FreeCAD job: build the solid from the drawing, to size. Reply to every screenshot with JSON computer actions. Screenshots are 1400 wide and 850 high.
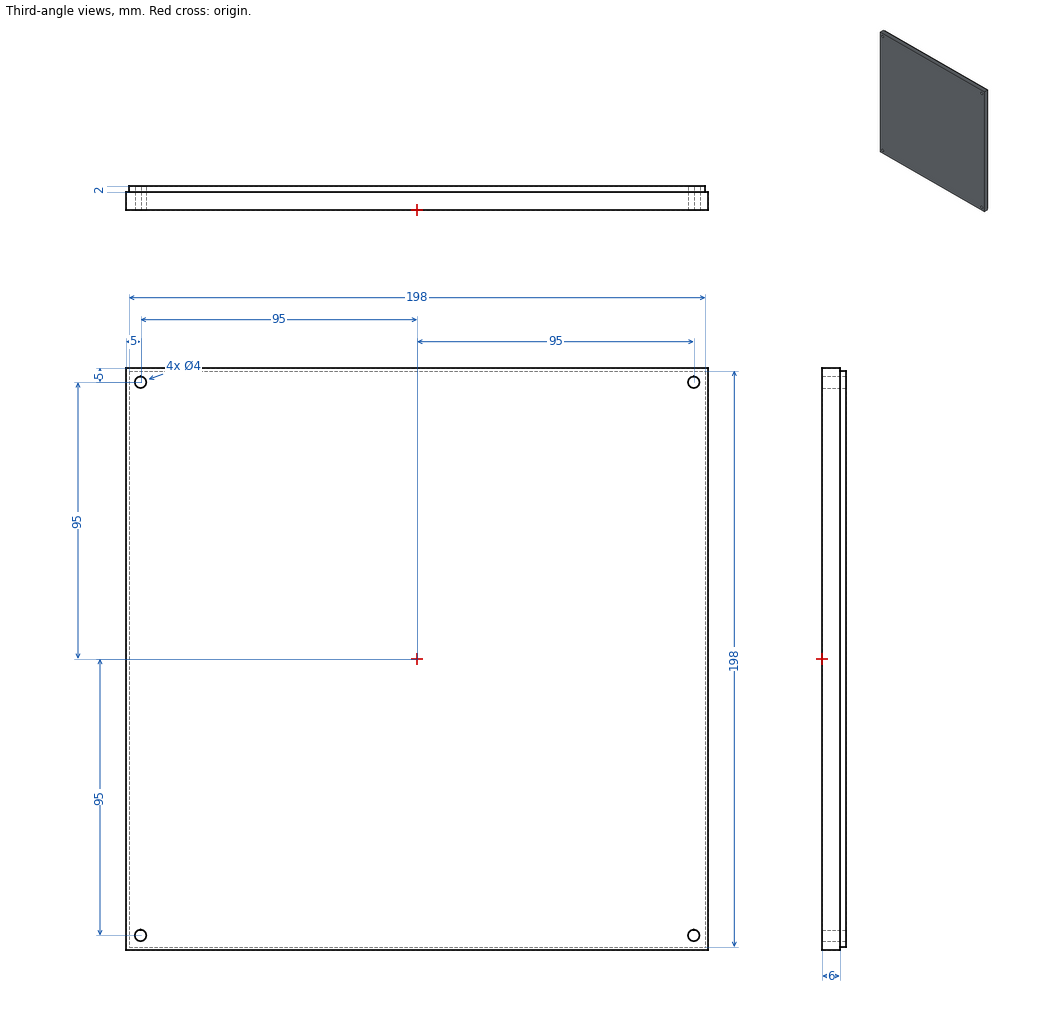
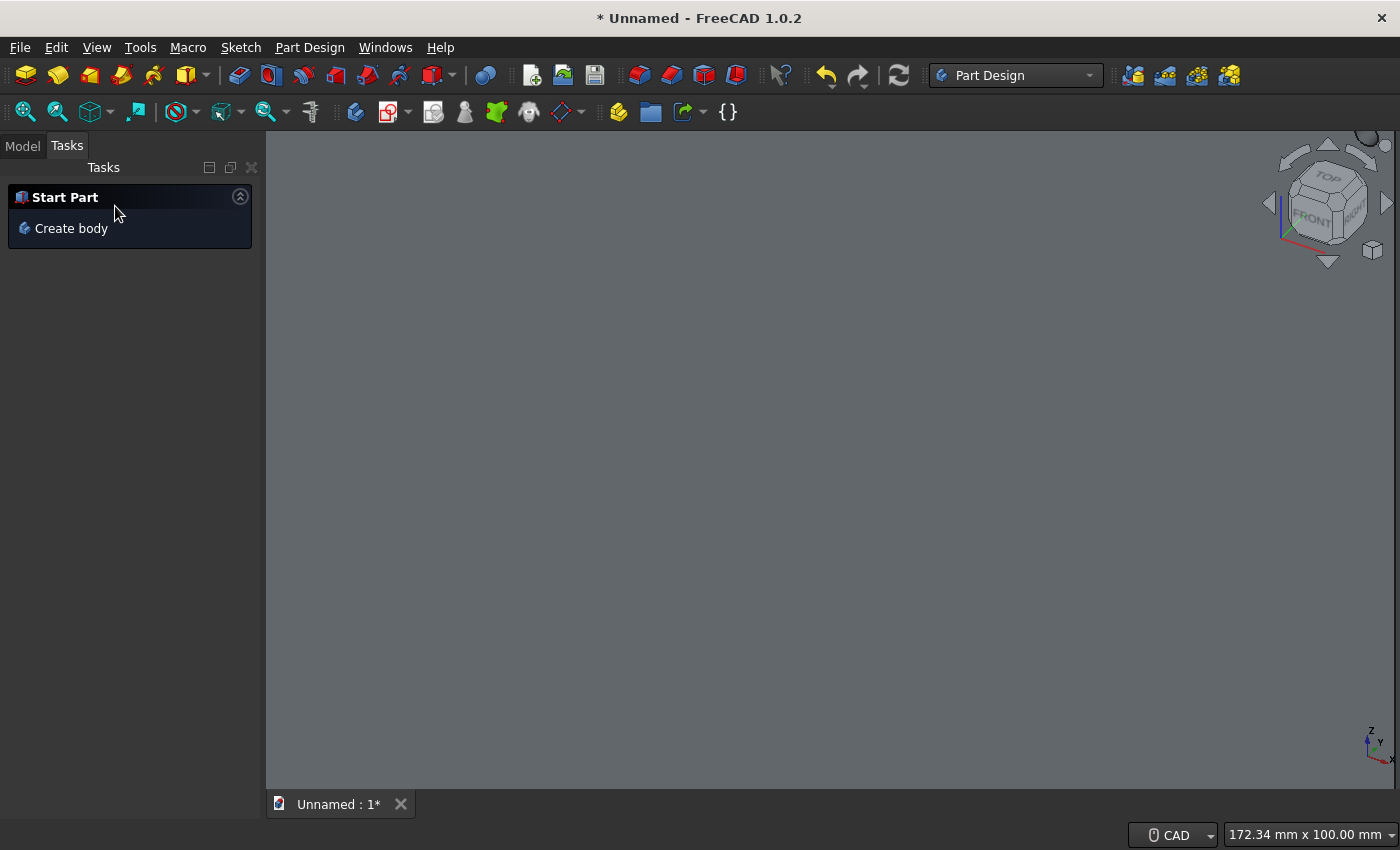
{"action": "left_click", "coordinate": [26, 112]}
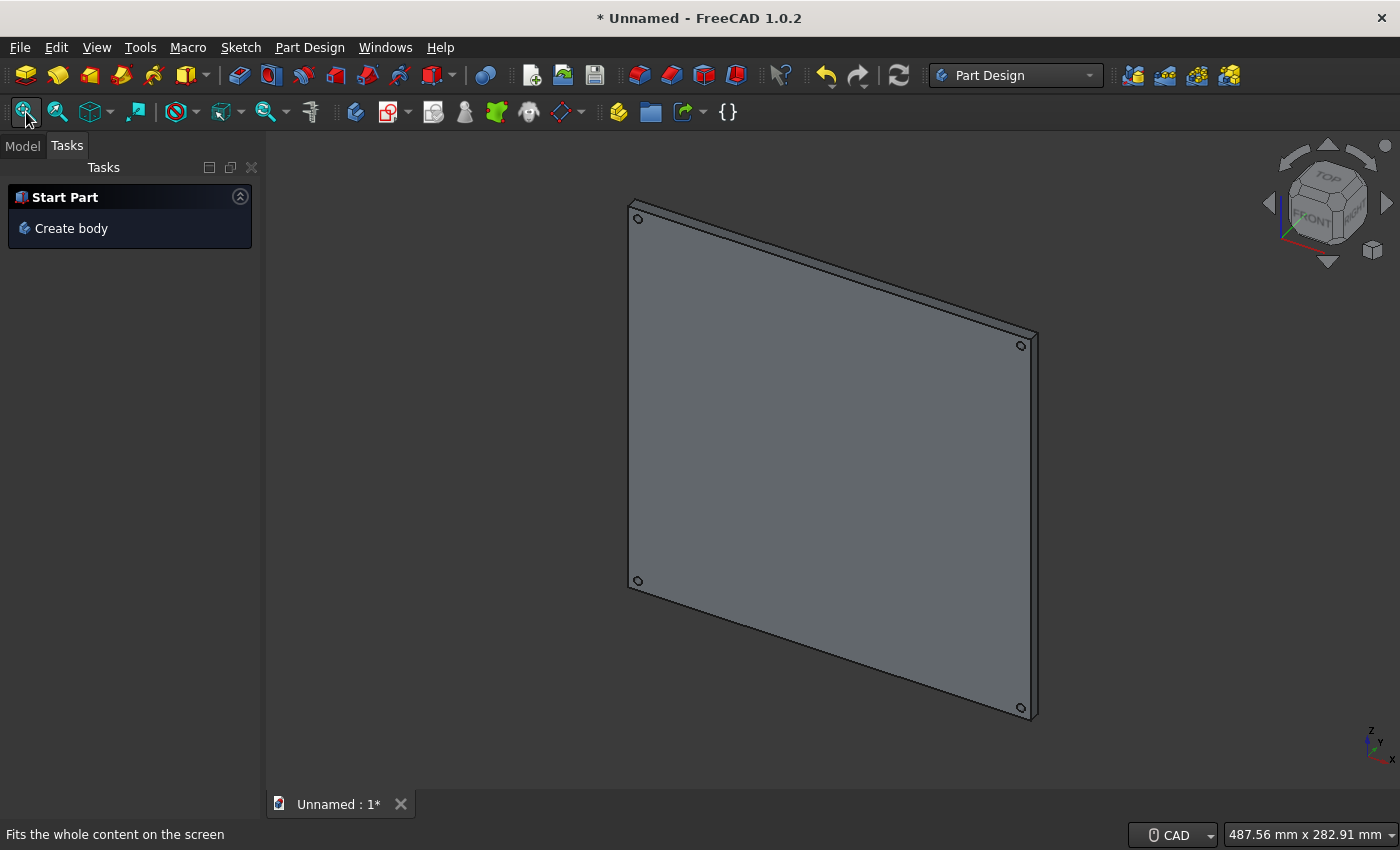
{"action": "key", "text": "4"}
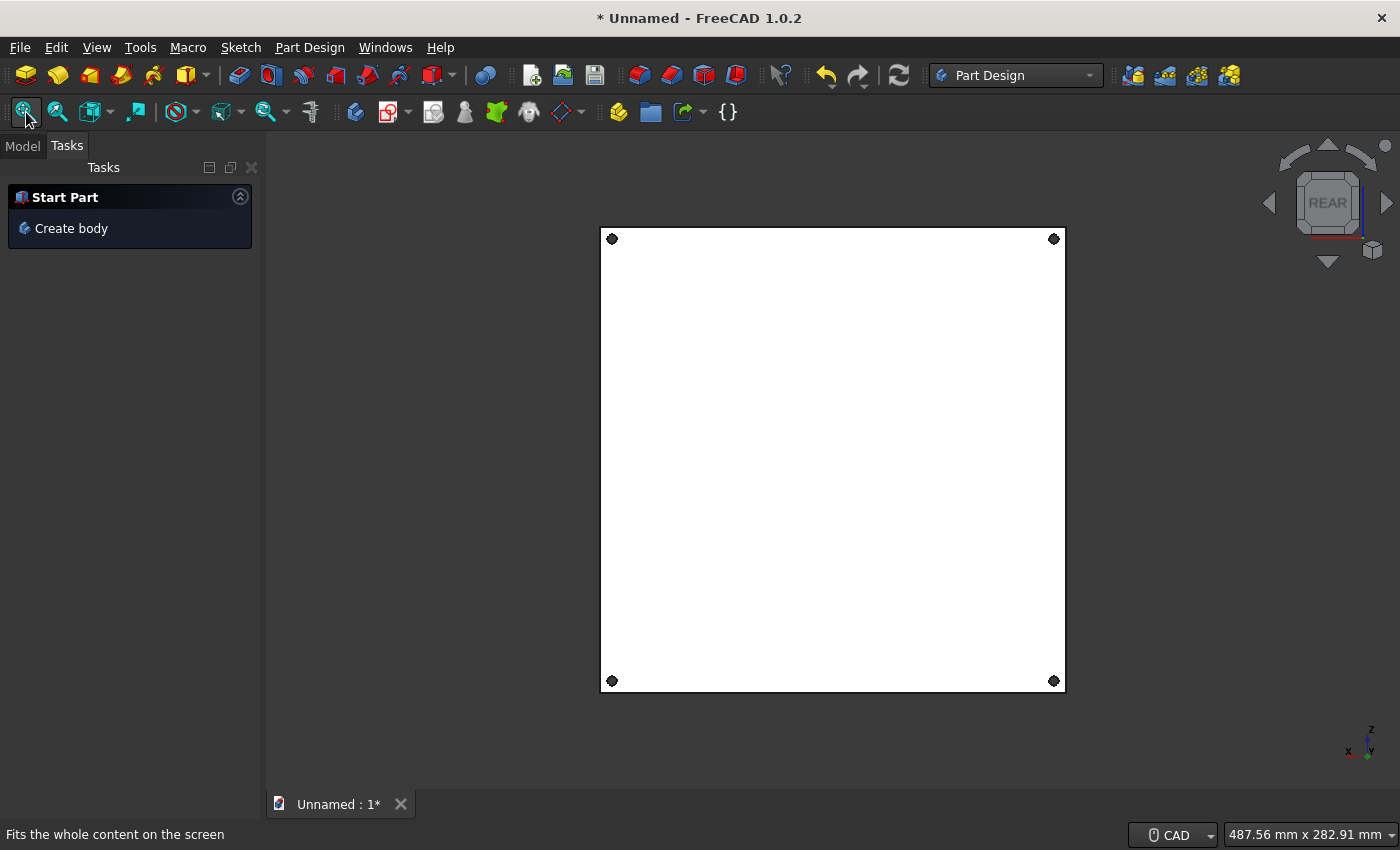
{"action": "left_click", "coordinate": [833, 459]}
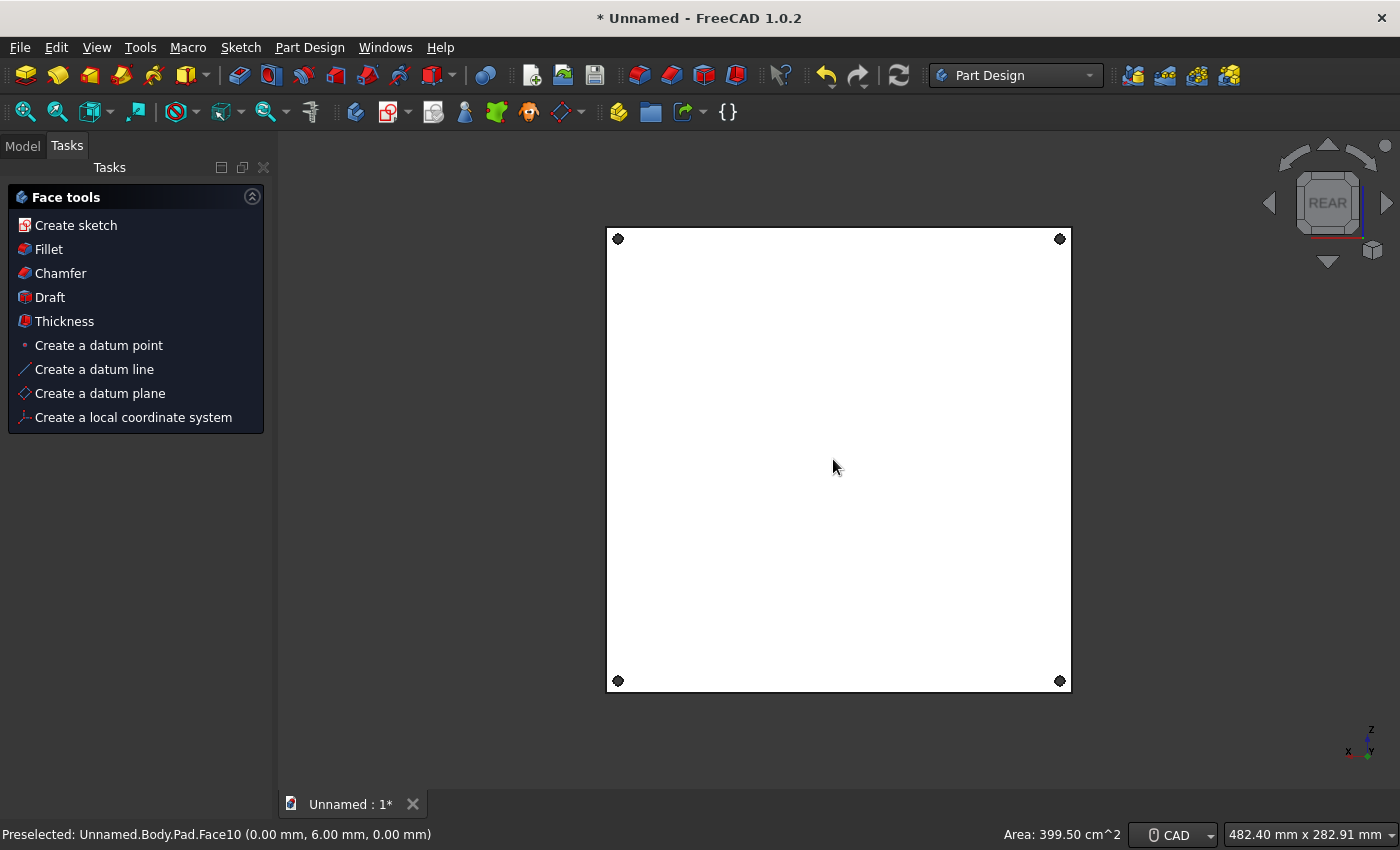
{"action": "left_click", "coordinate": [388, 112]}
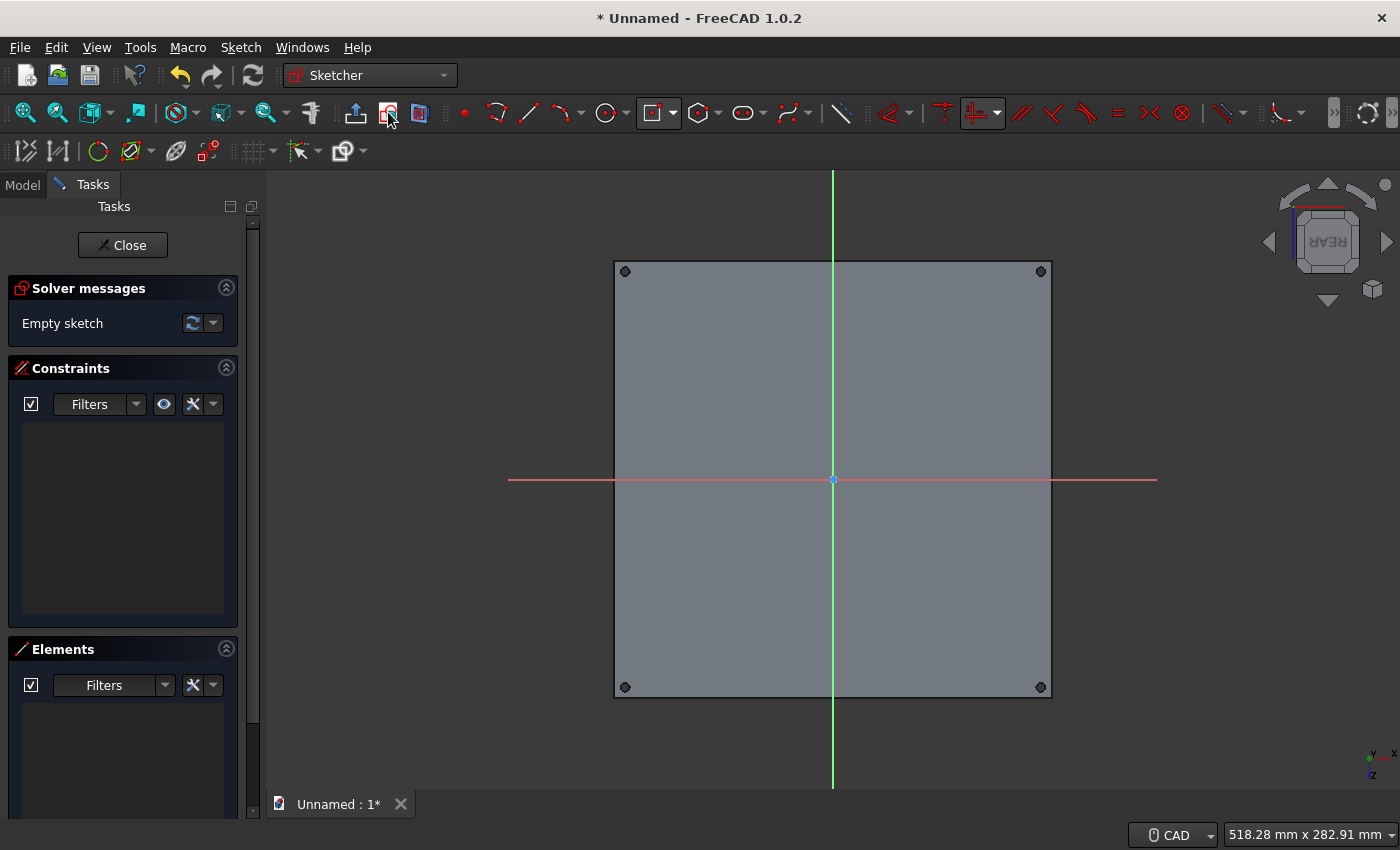
{"action": "left_click", "coordinate": [652, 114]}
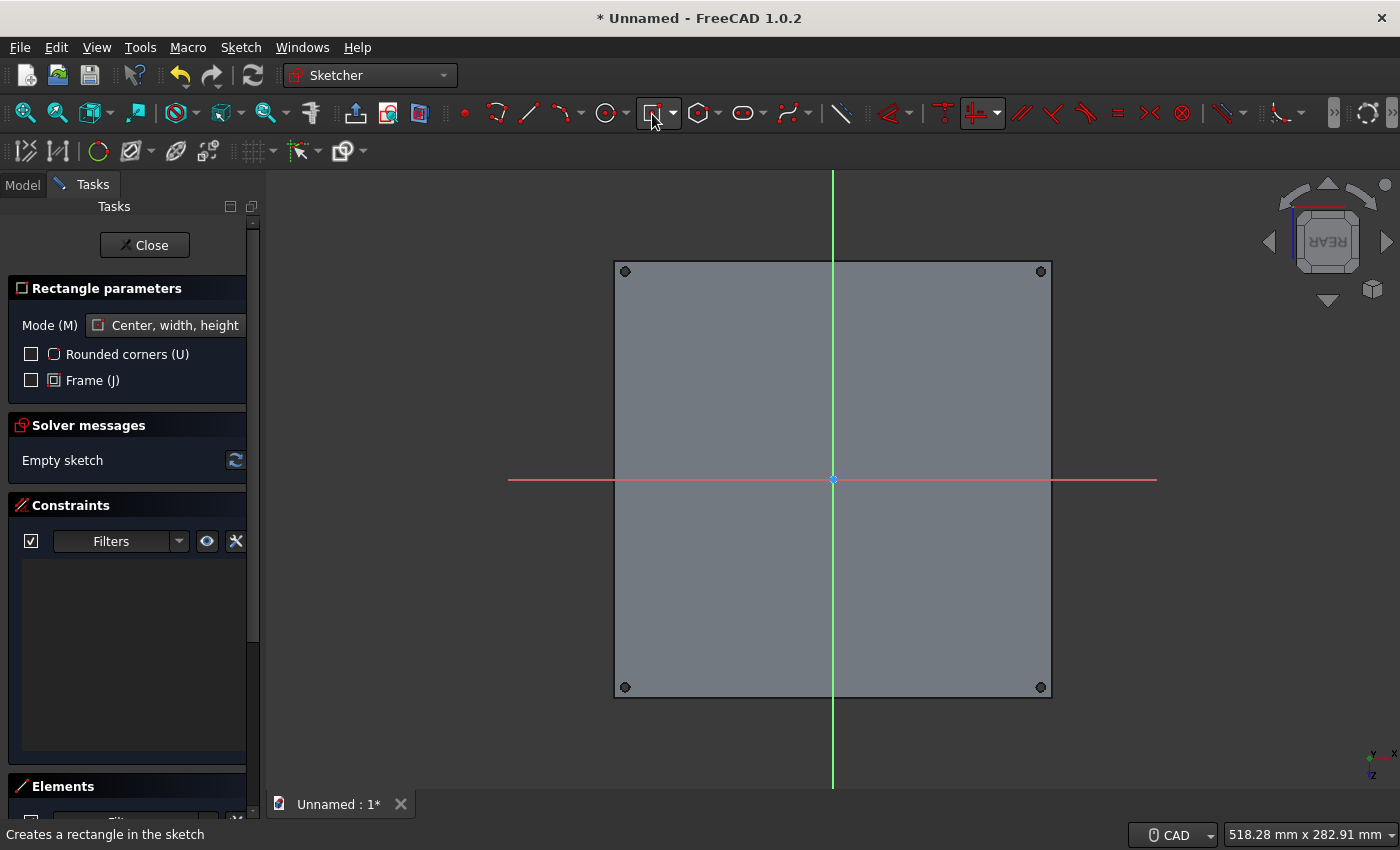
{"action": "left_click", "coordinate": [833, 480]}
{"action": "left_click", "coordinate": [1050, 263]}
{"action": "key", "text": "Escape"}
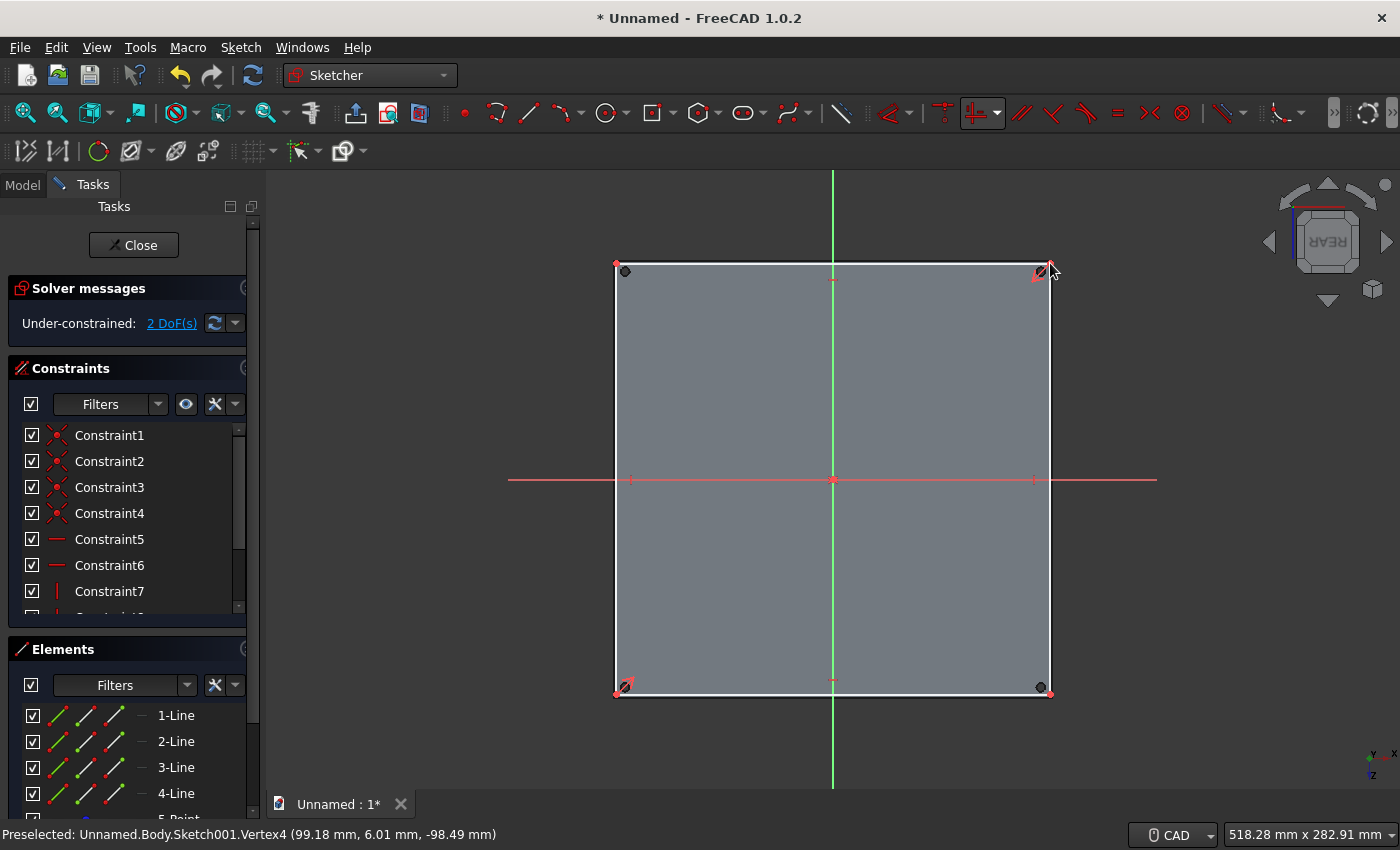
{"action": "left_click", "coordinate": [888, 114]}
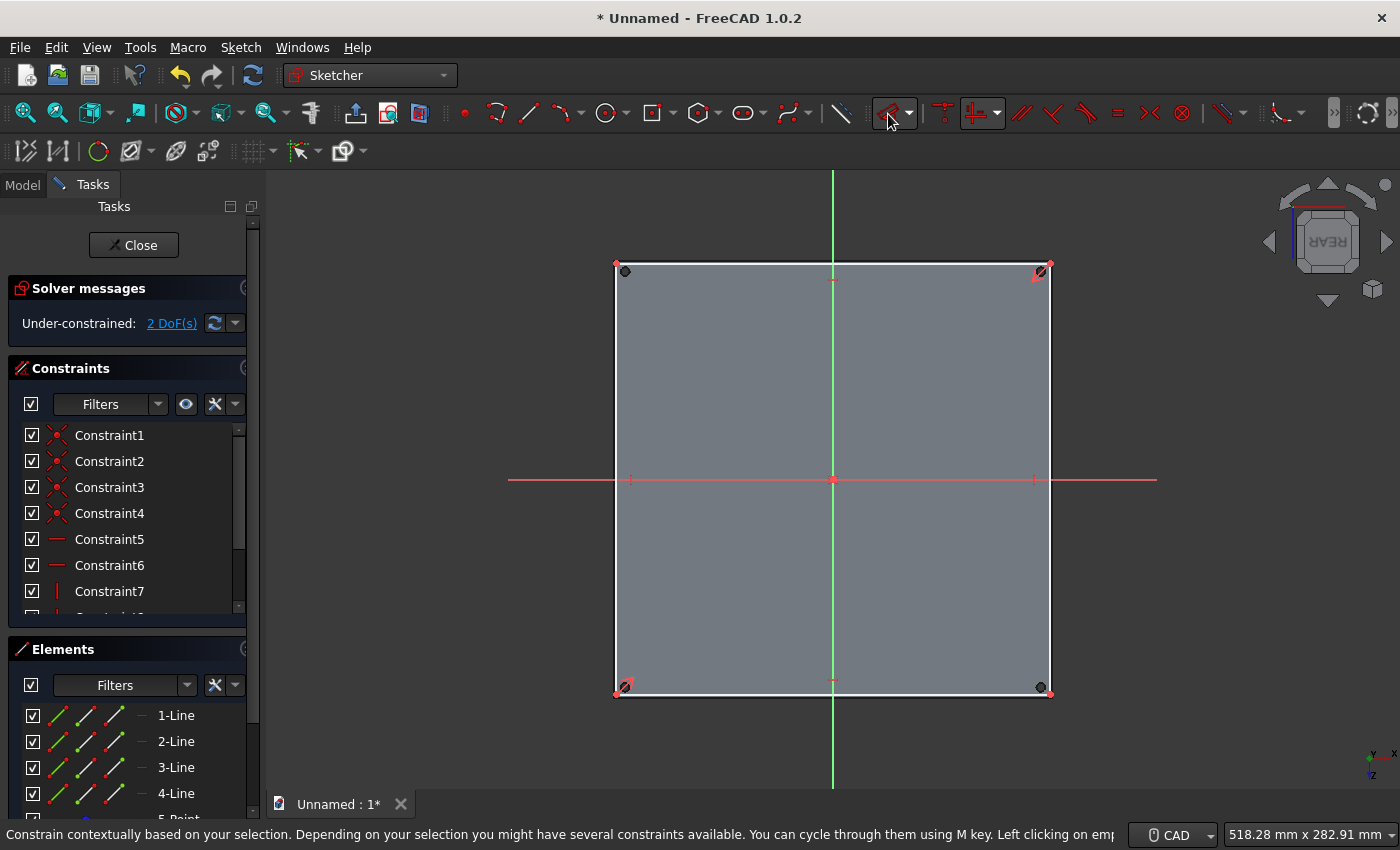
{"action": "left_click", "coordinate": [746, 695]}
{"action": "left_click", "coordinate": [733, 729]}